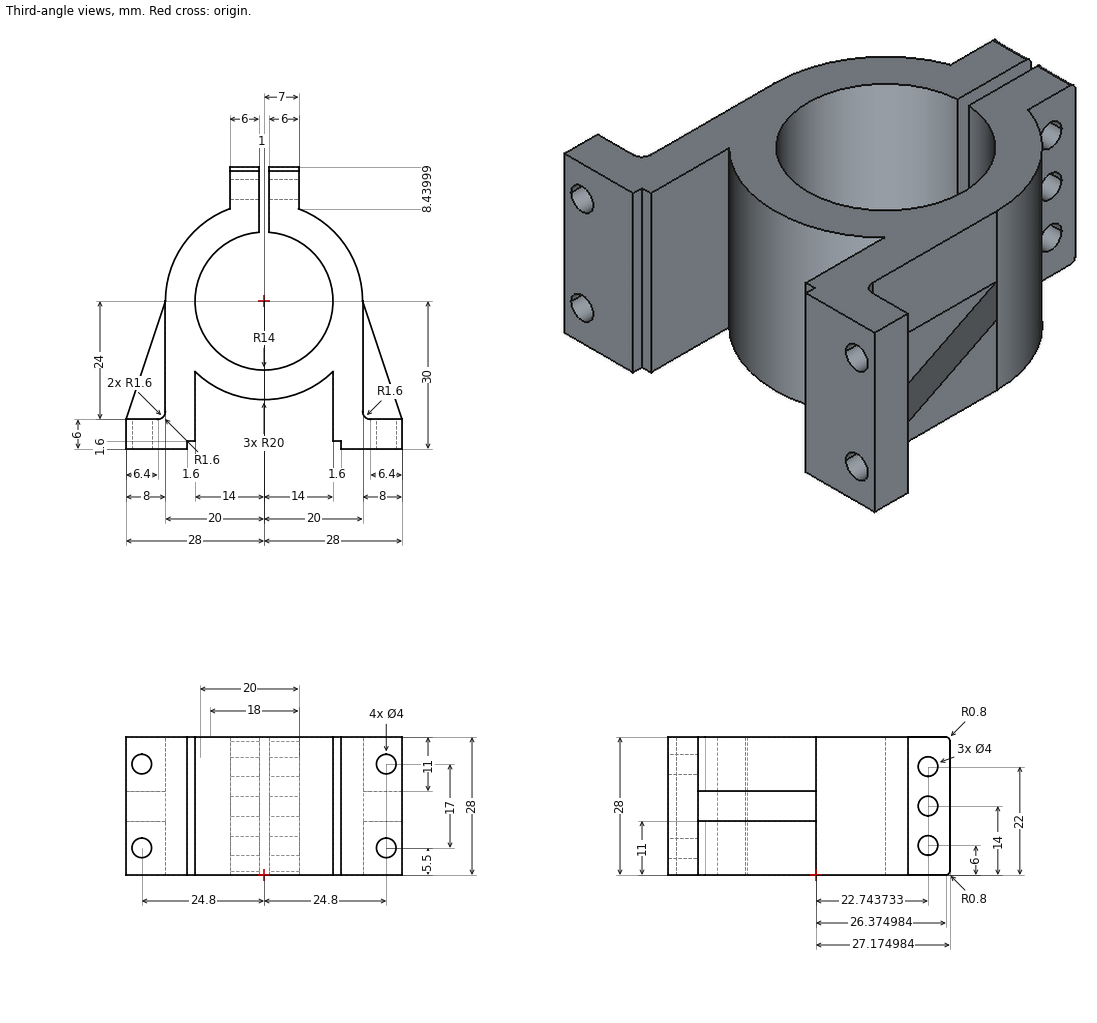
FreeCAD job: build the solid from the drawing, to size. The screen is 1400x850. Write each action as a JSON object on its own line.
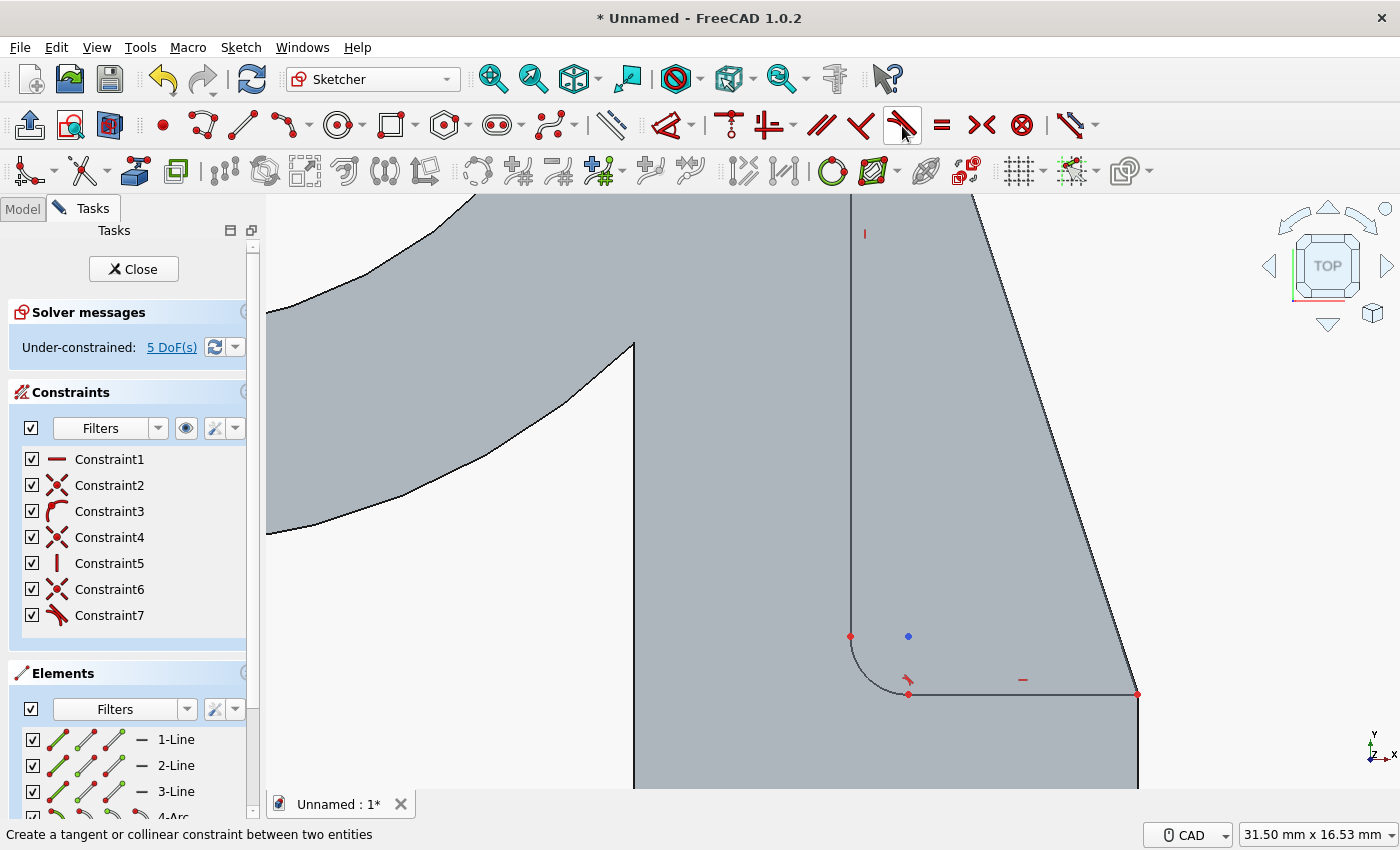
{"action": "left_click", "coordinate": [851, 395]}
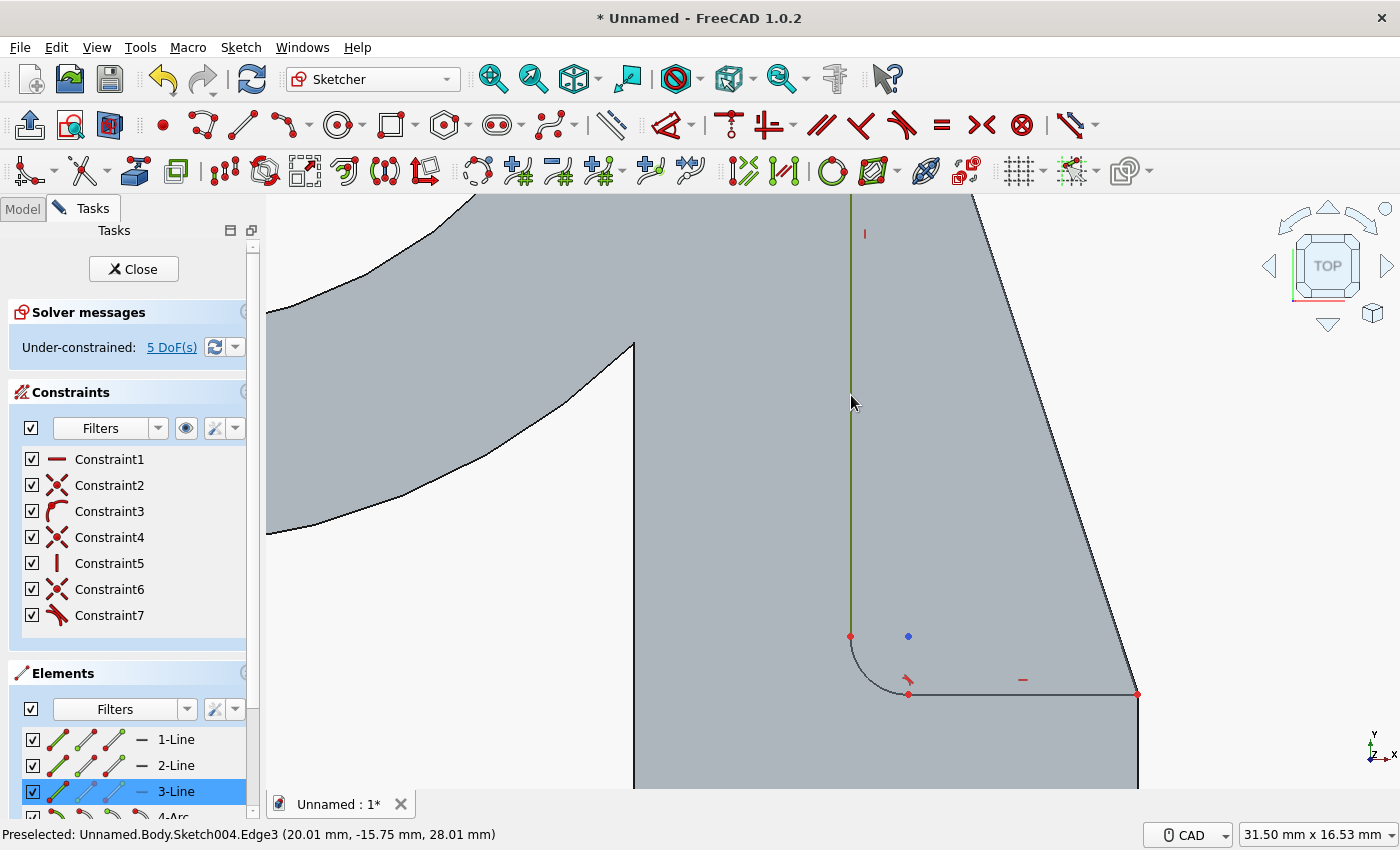
{"action": "left_click", "coordinate": [857, 663]}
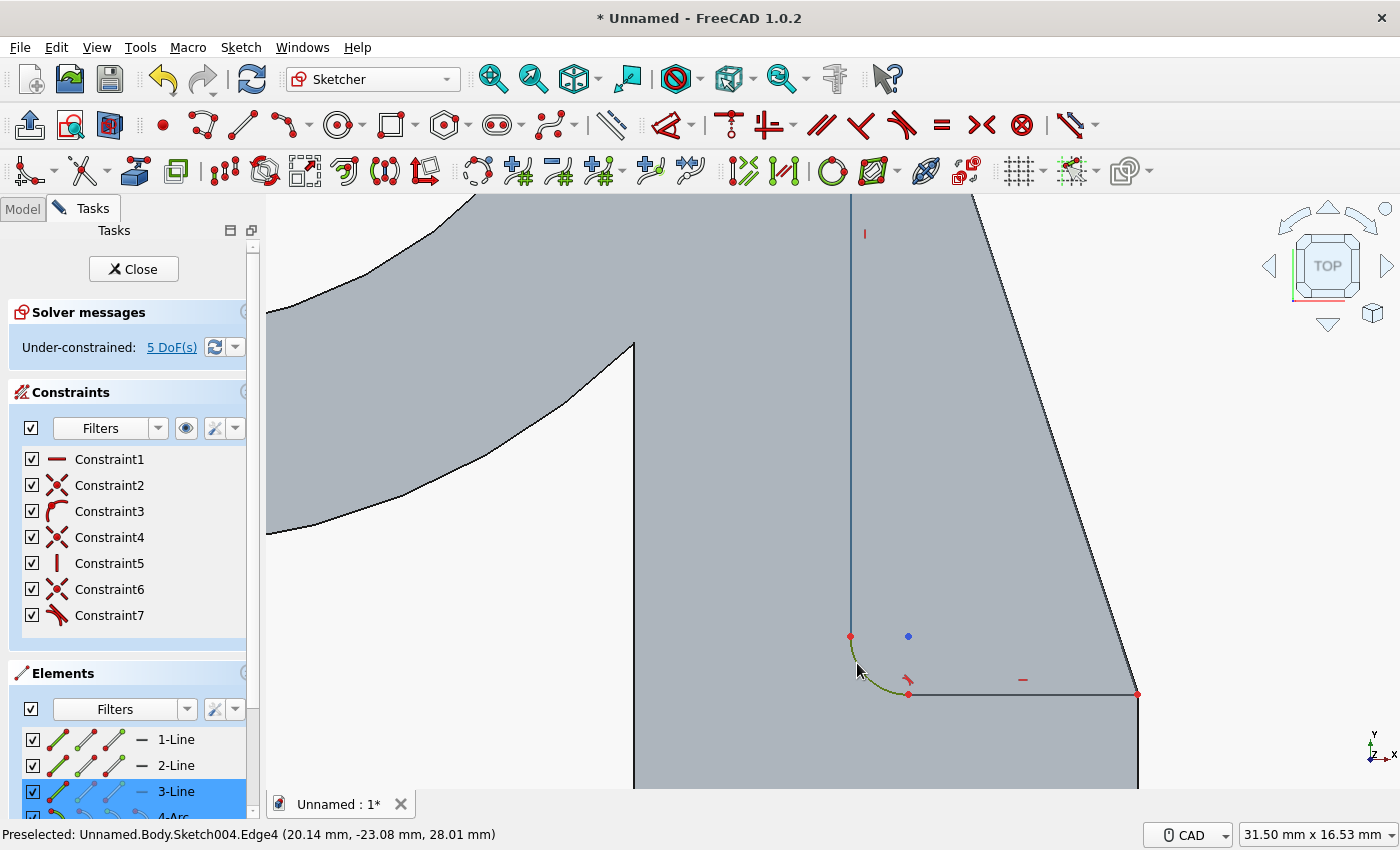
{"action": "left_click", "coordinate": [902, 126]}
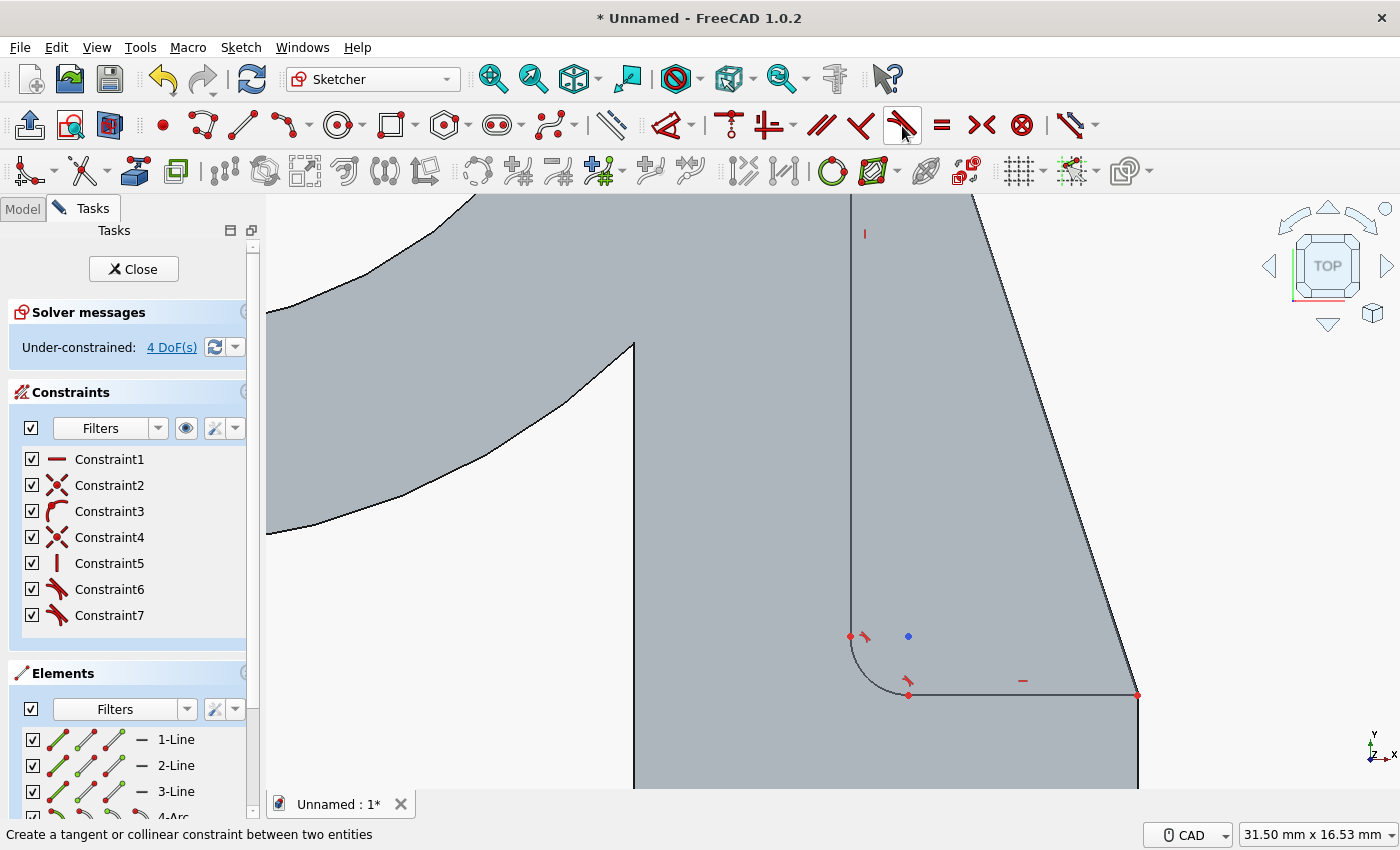
{"action": "left_click", "coordinate": [666, 126]}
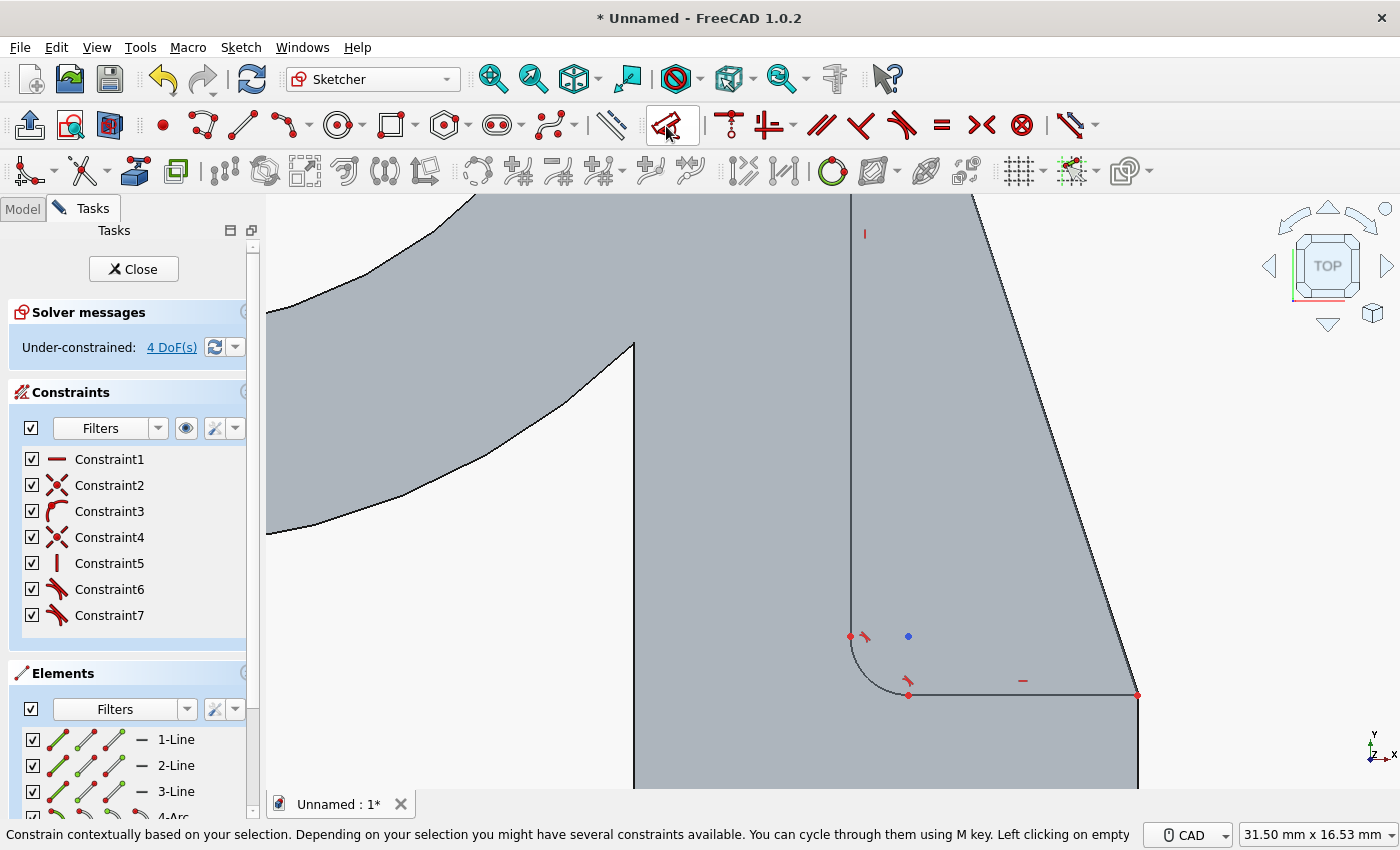
{"action": "left_click", "coordinate": [857, 663]}
{"action": "left_click", "coordinate": [828, 677]}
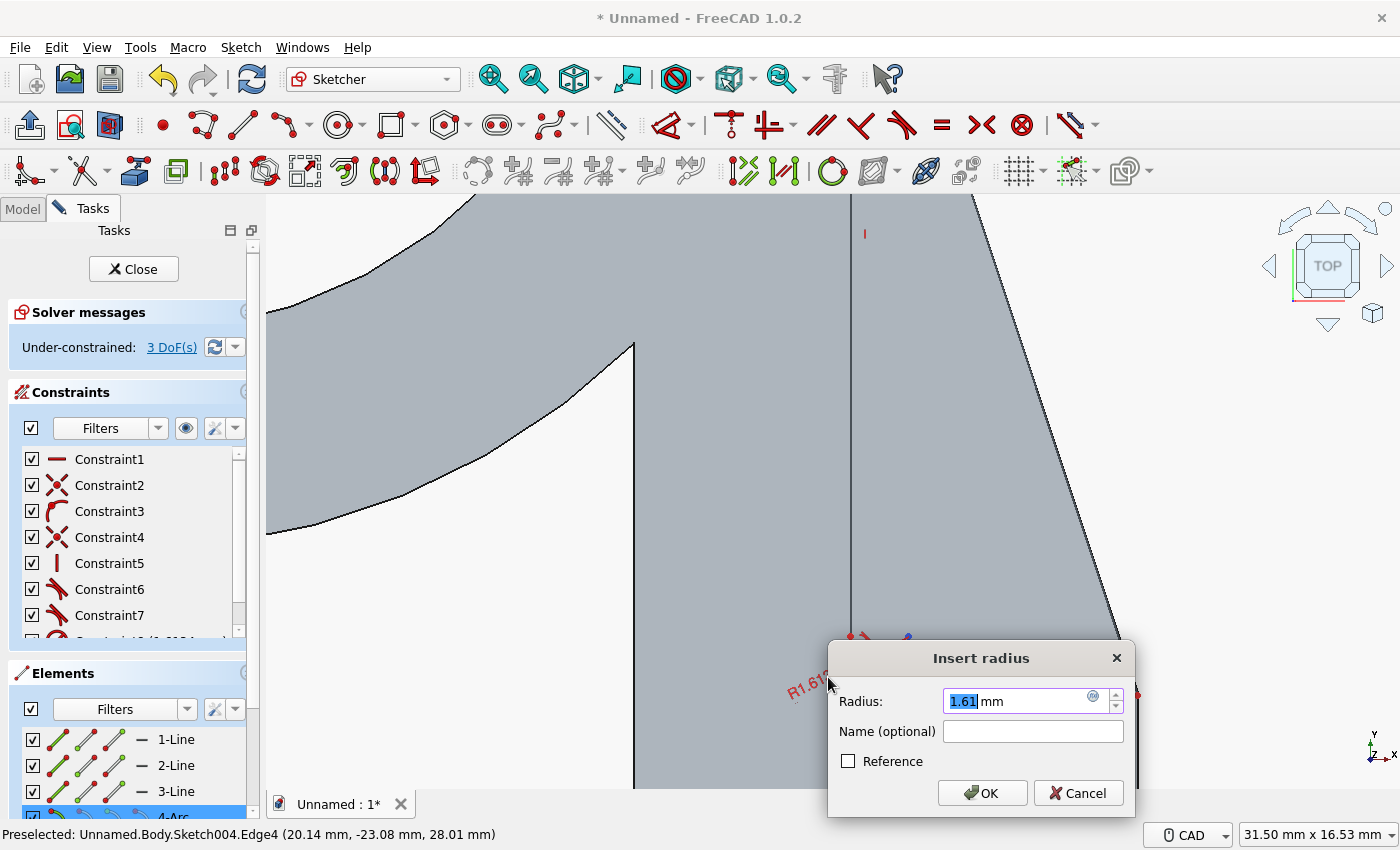
{"action": "type", "text": "1.6"}
{"action": "key", "text": "Return"}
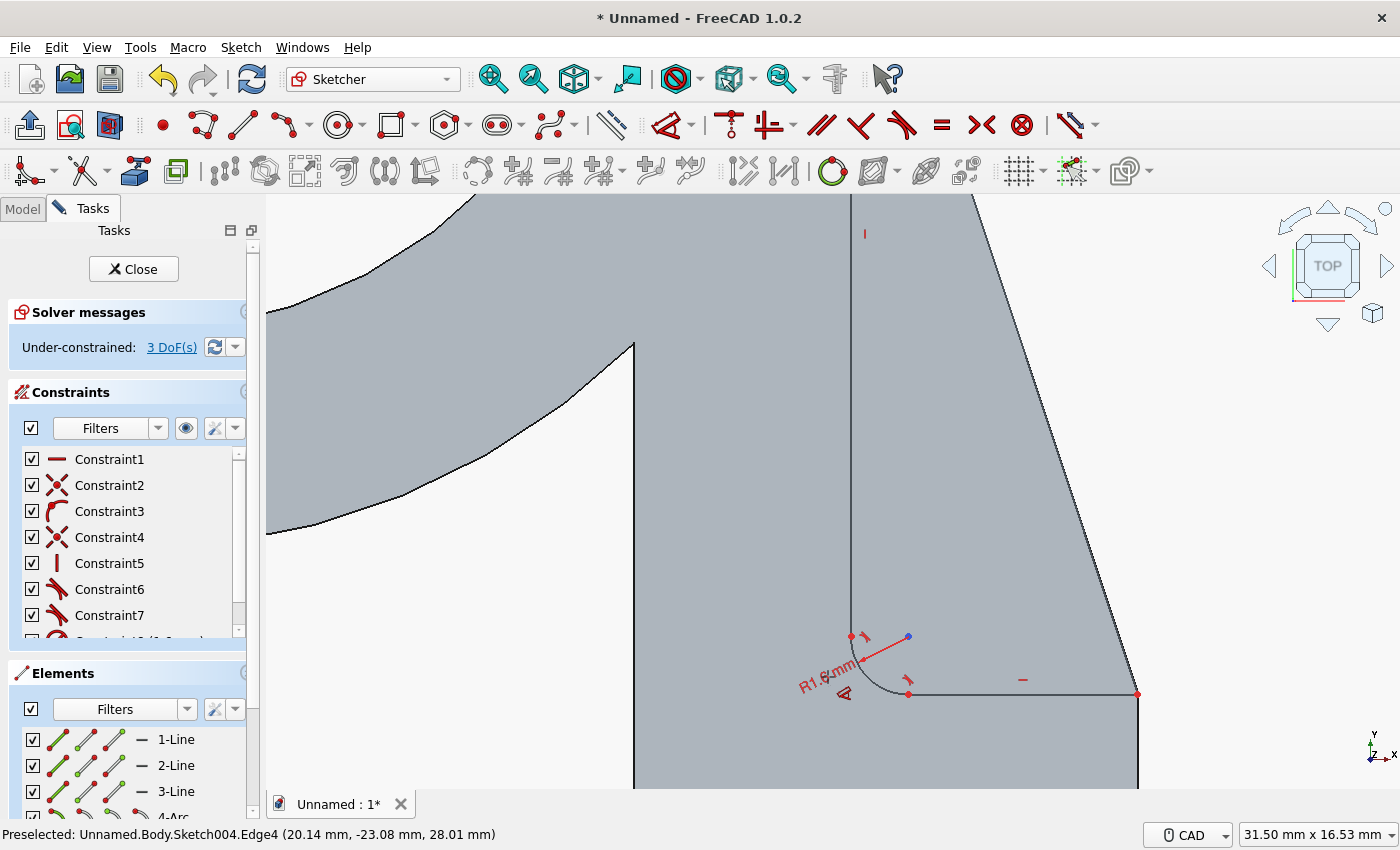
{"action": "left_click", "coordinate": [1052, 435]}
{"action": "left_click", "coordinate": [994, 729]}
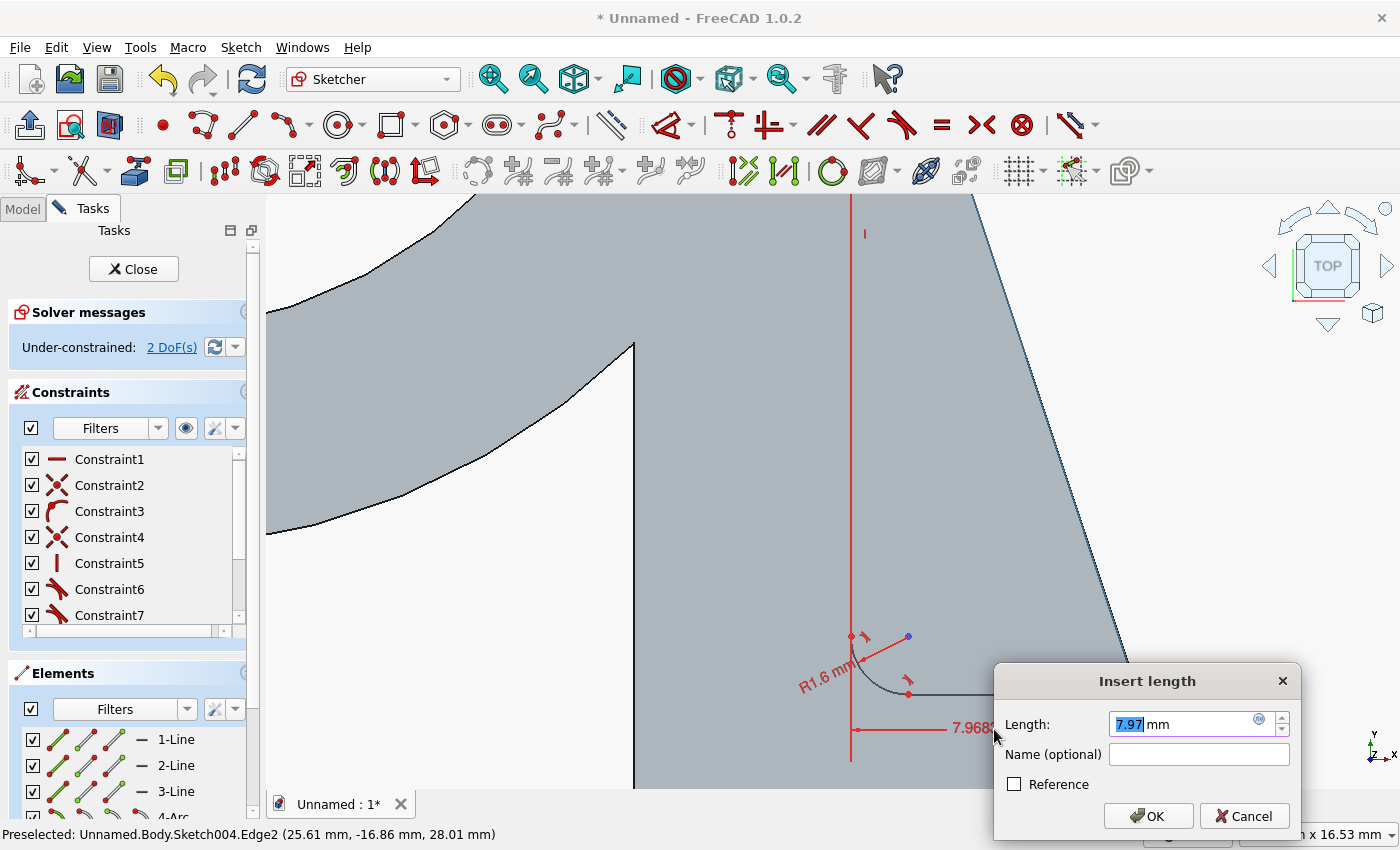
{"action": "type", "text": "8"}
{"action": "key", "text": "Return"}